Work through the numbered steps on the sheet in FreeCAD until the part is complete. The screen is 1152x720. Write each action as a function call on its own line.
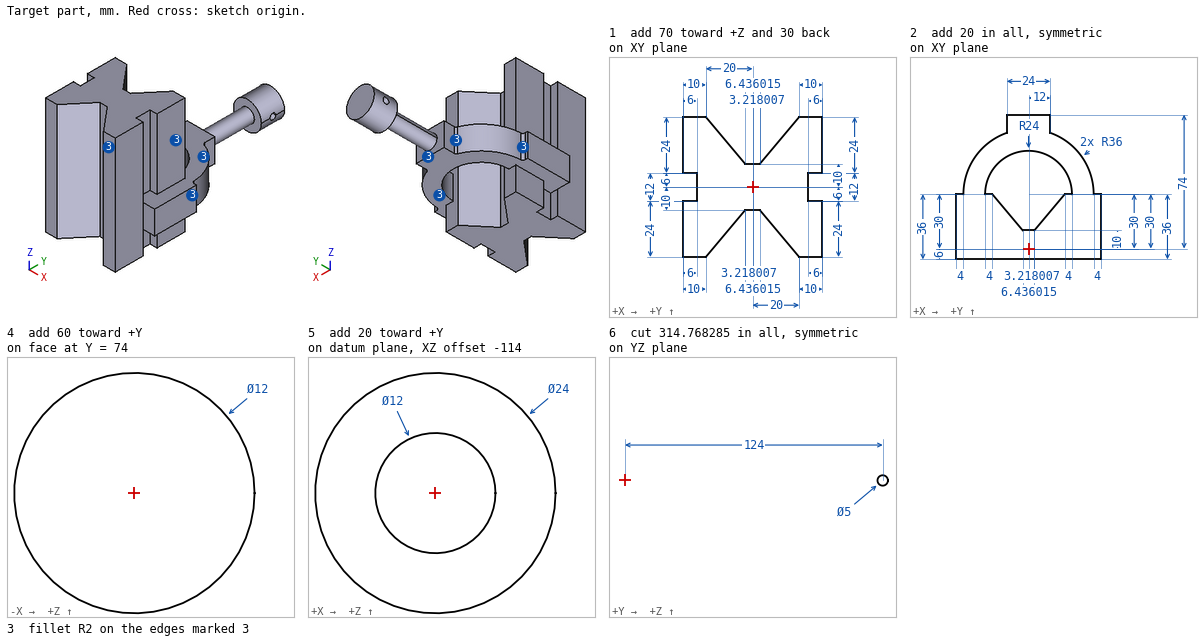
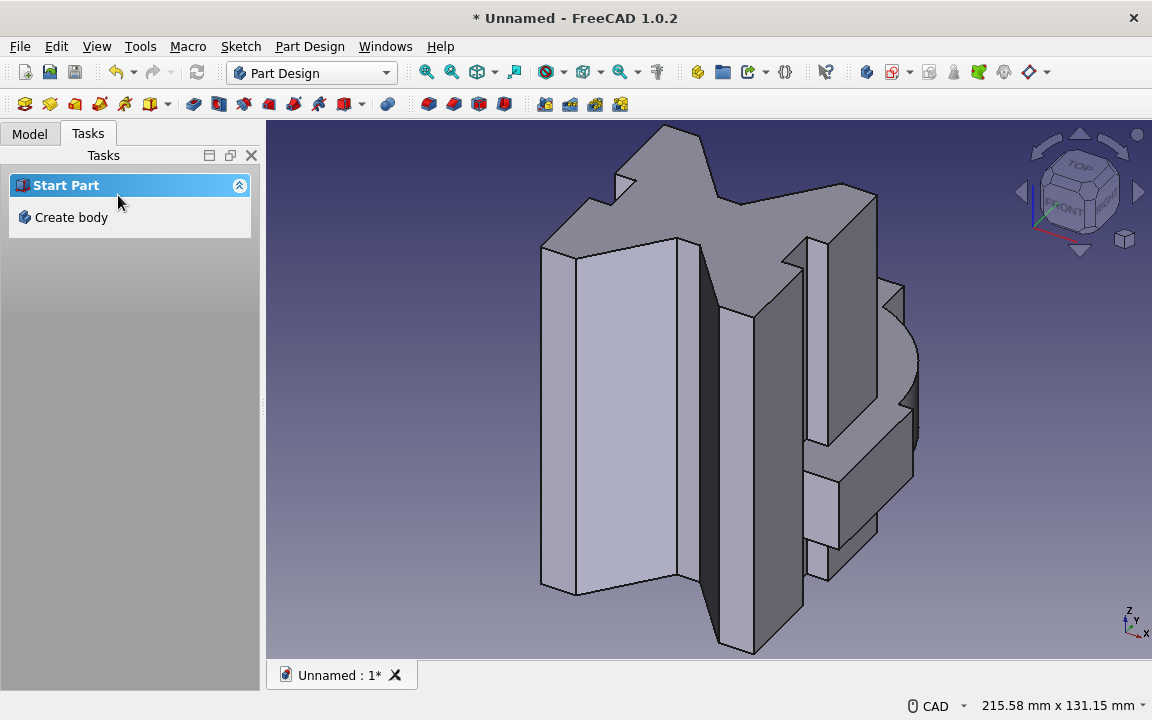
click(427, 72)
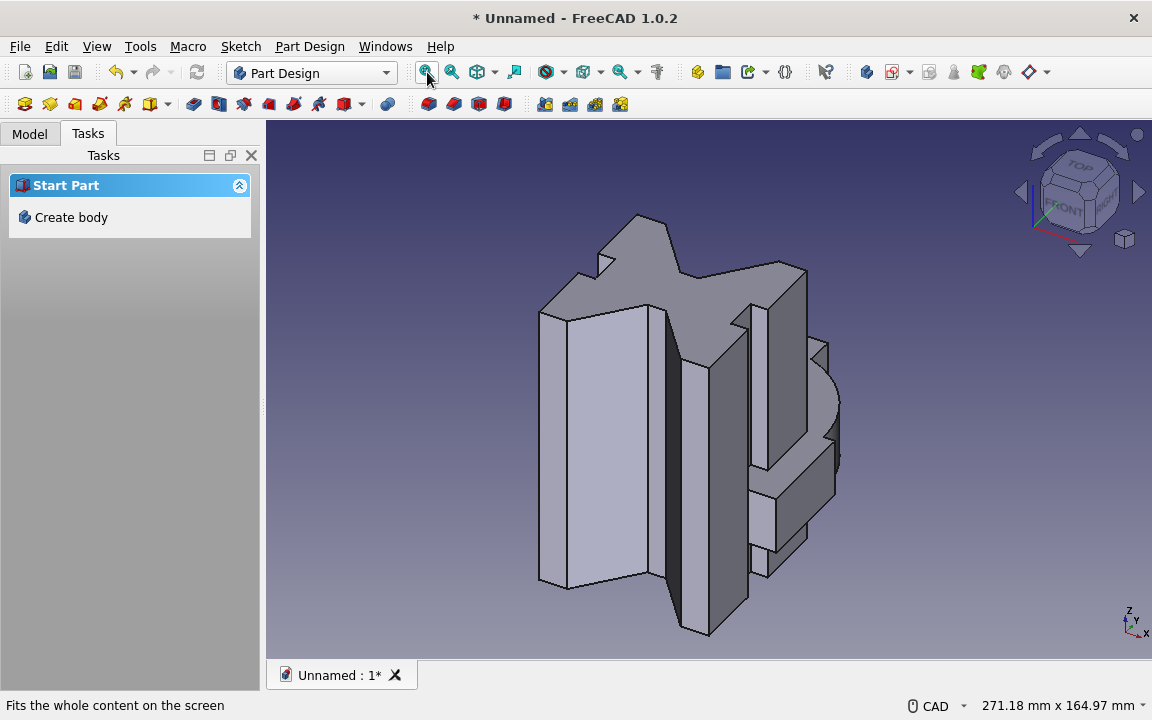
key(0)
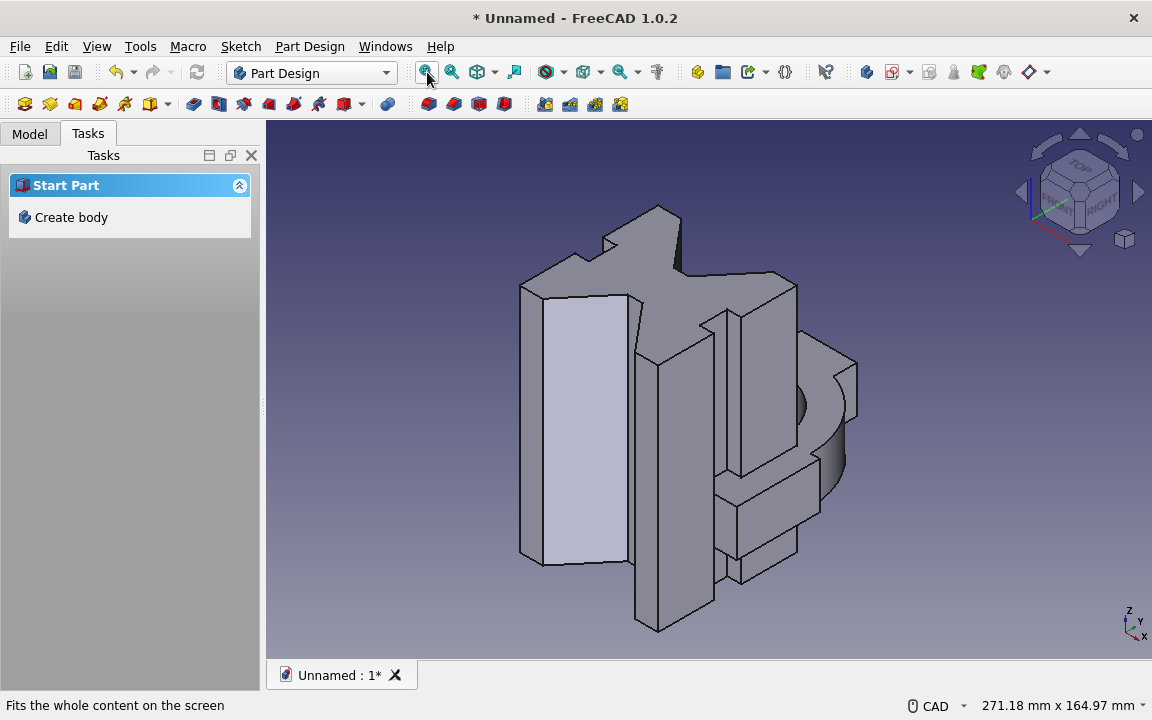
key(2)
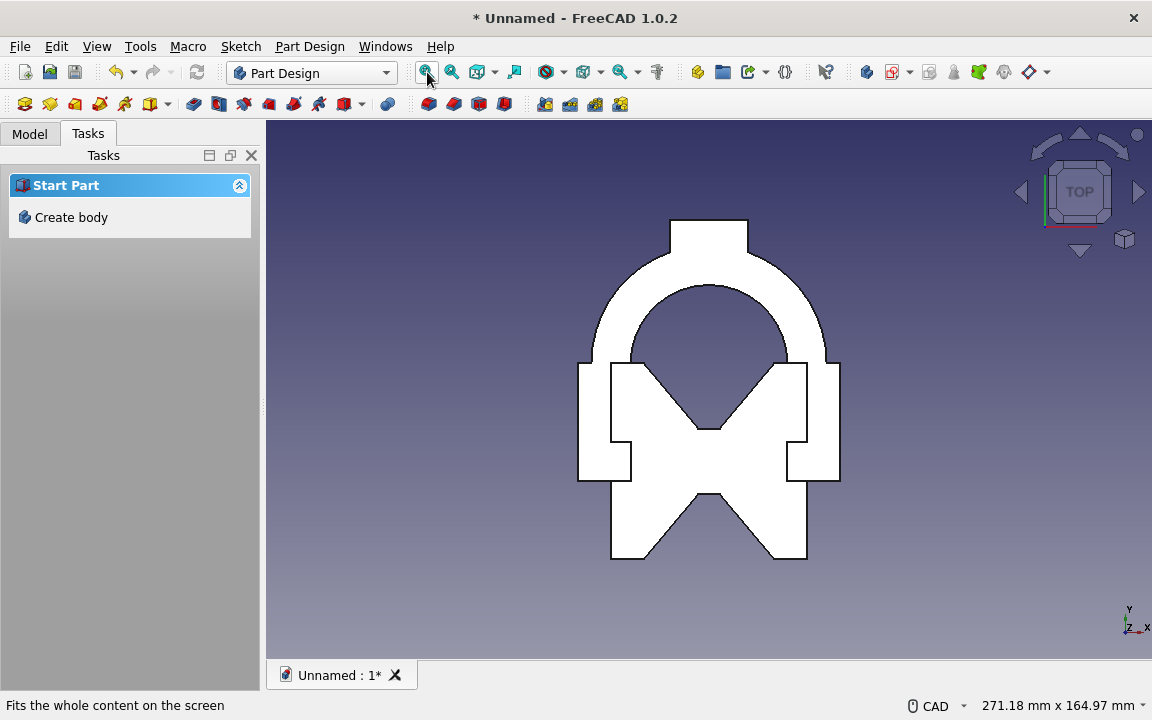
key(1)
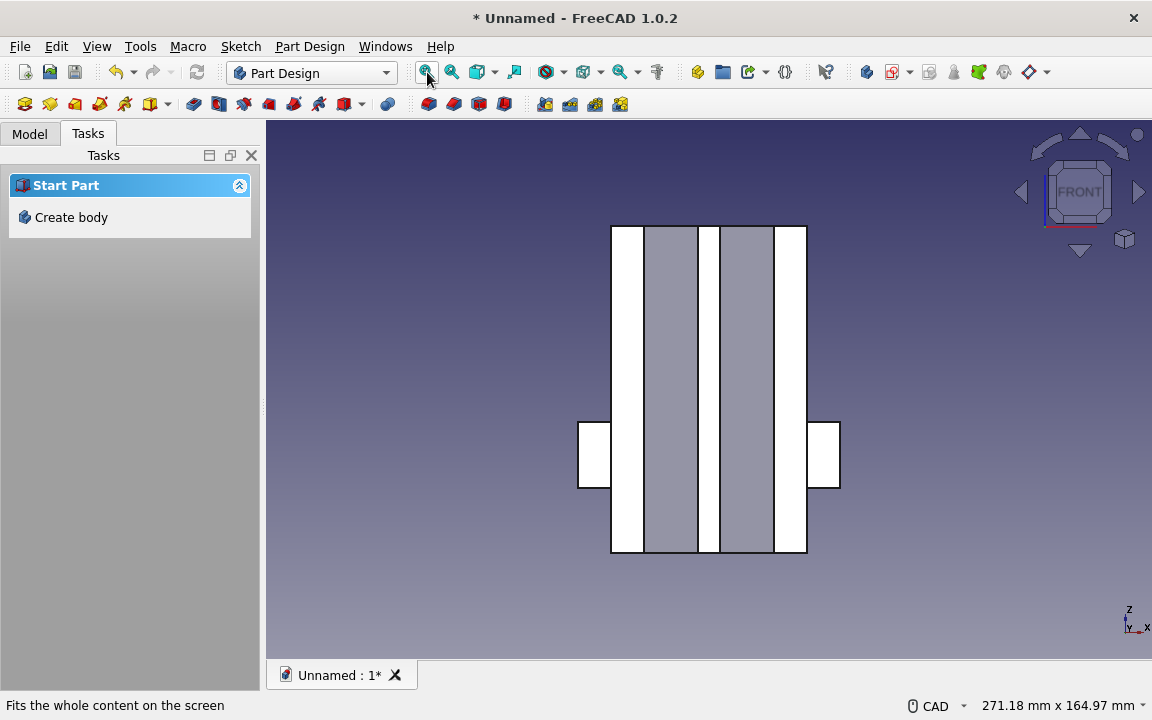
key(3)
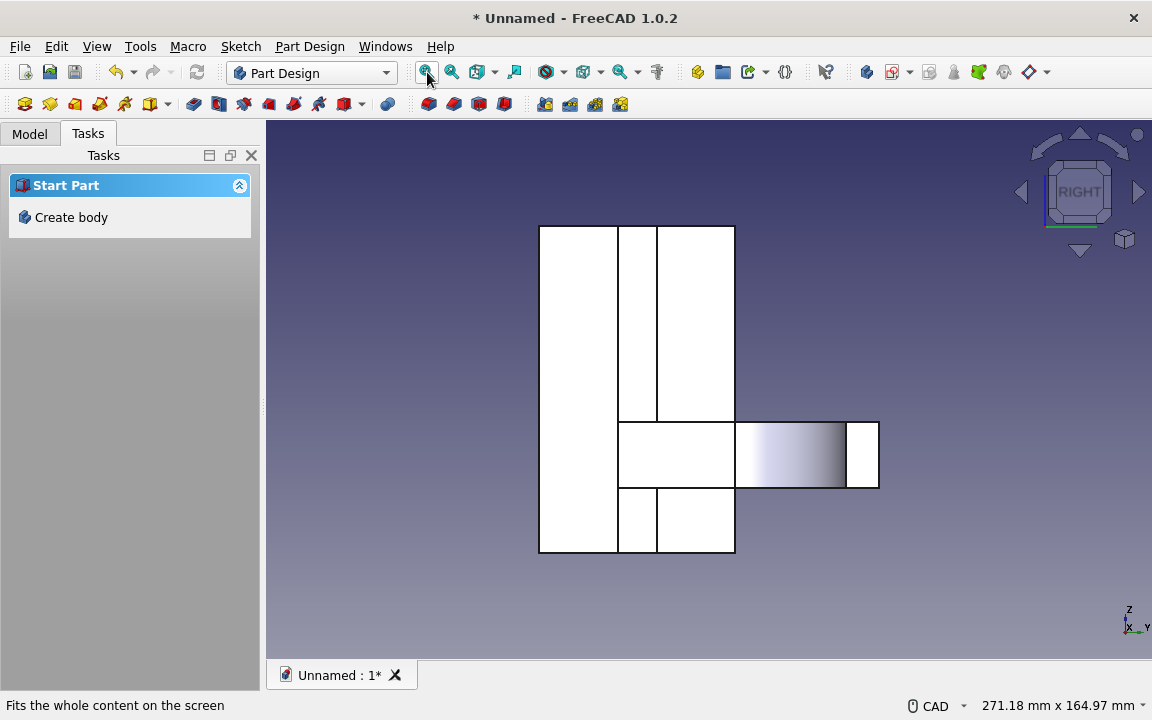
key(5)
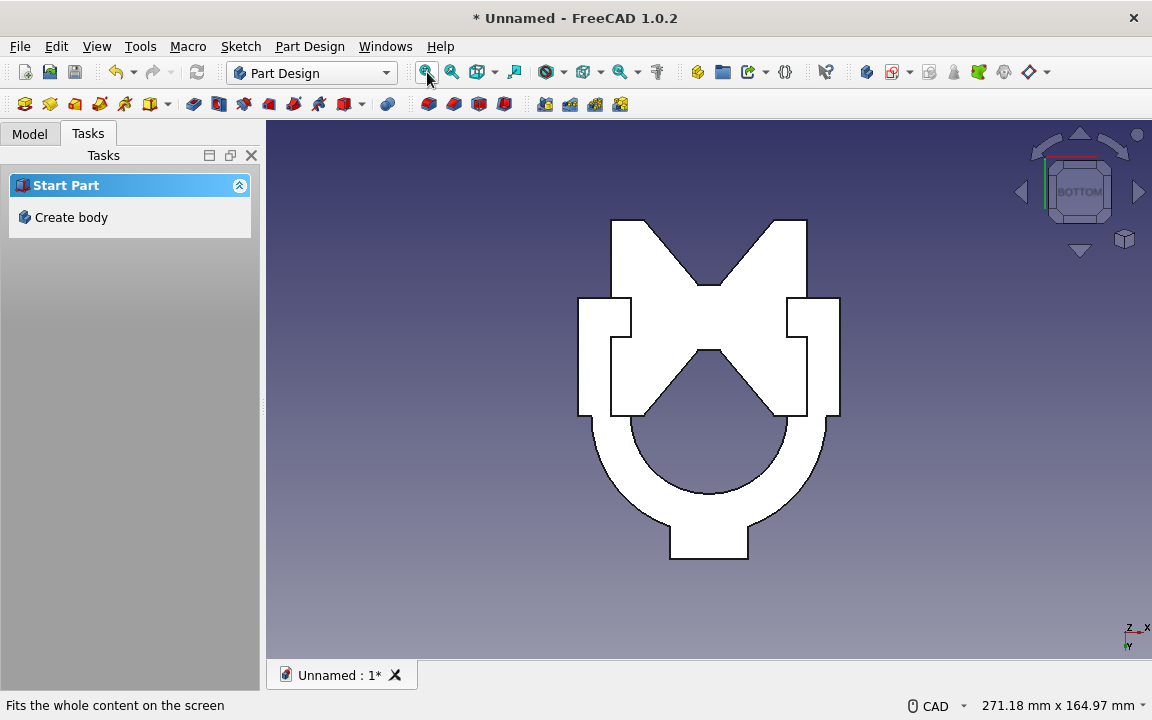
key(4)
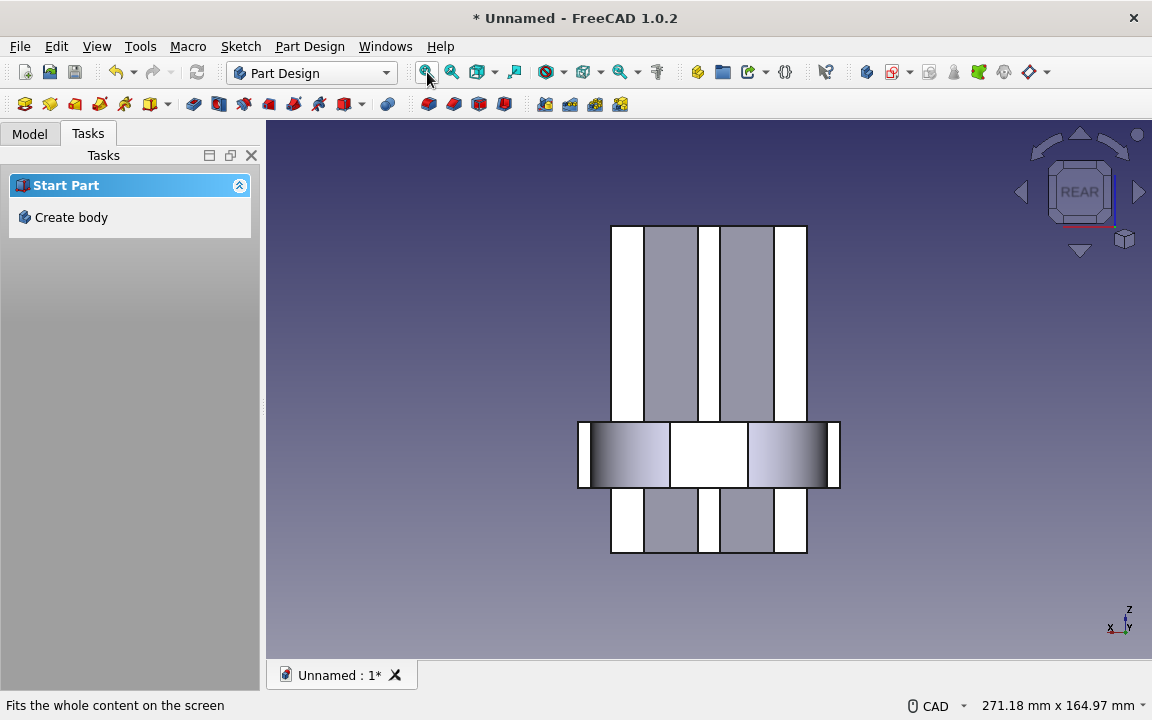
key(6)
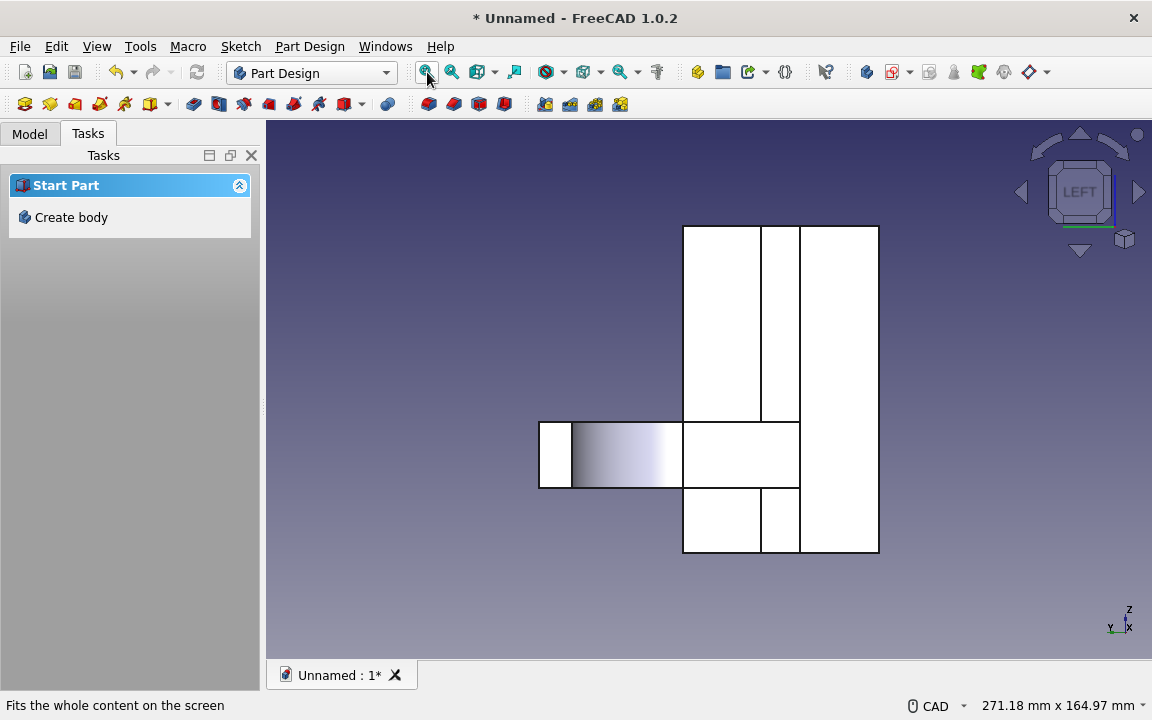
key(v)
key(3)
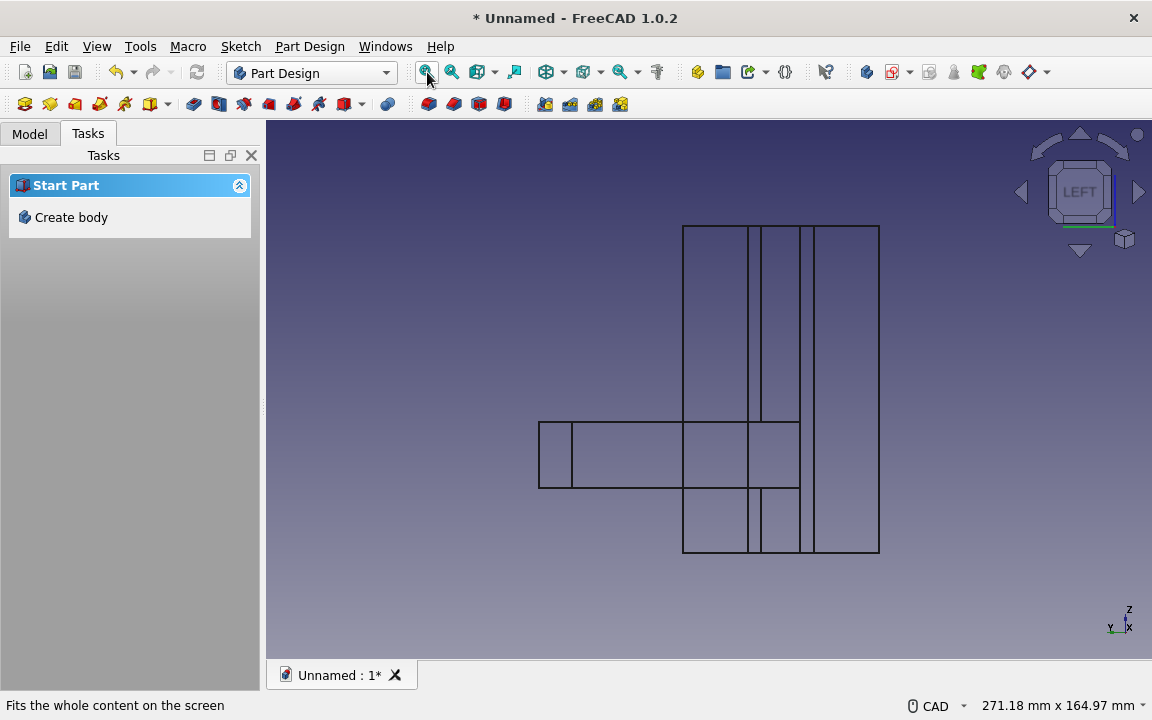
key(0)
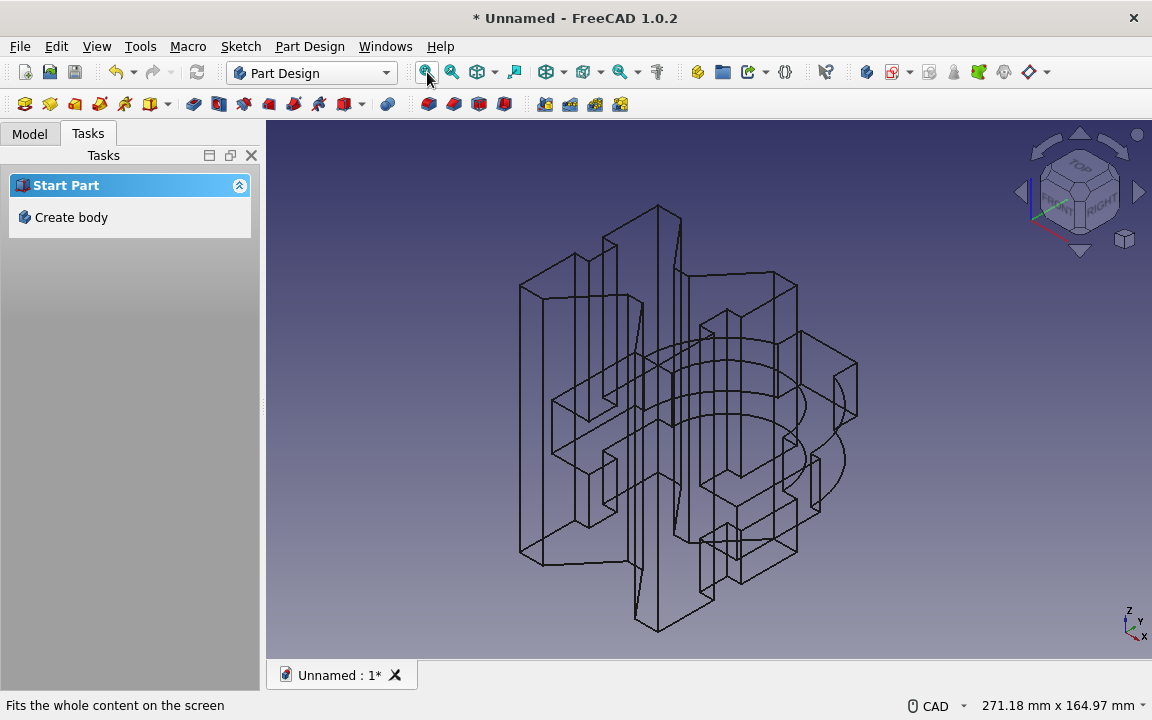
click(811, 479)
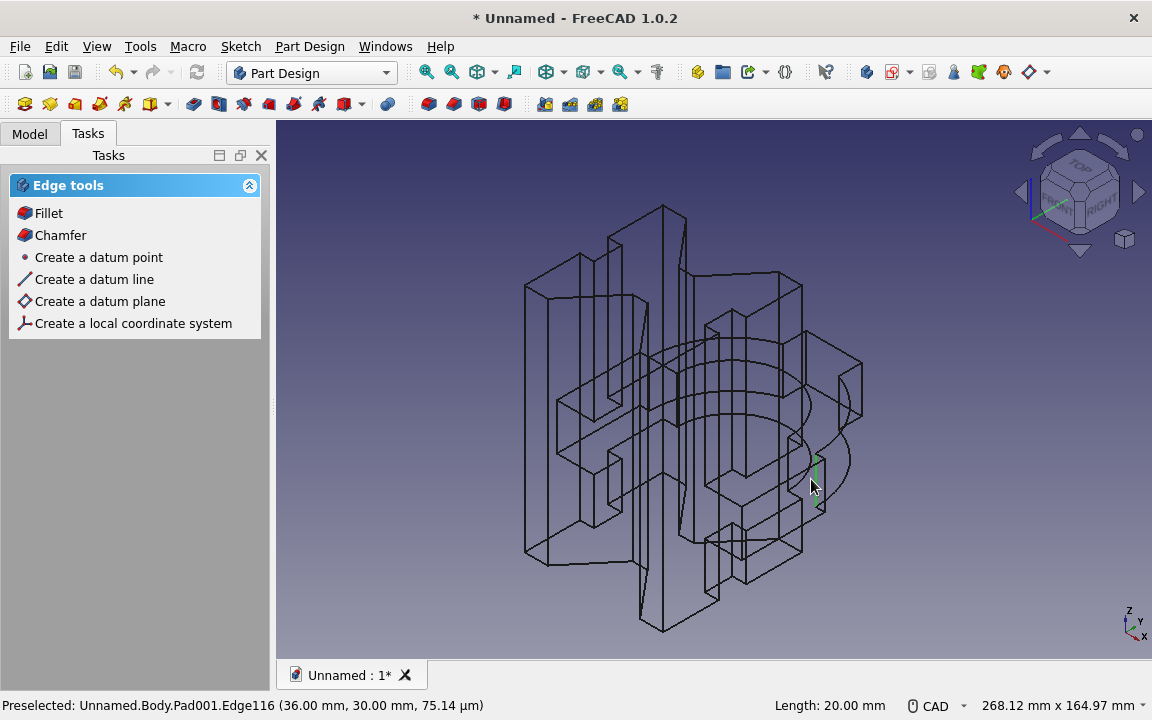
click(839, 402, ctrl)